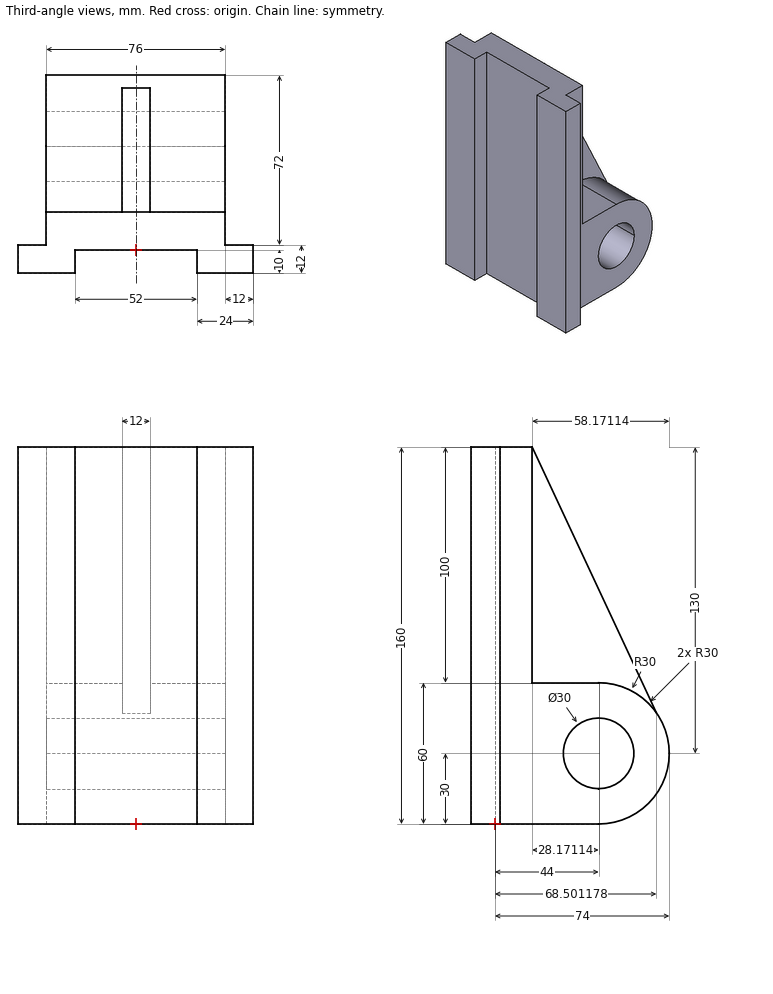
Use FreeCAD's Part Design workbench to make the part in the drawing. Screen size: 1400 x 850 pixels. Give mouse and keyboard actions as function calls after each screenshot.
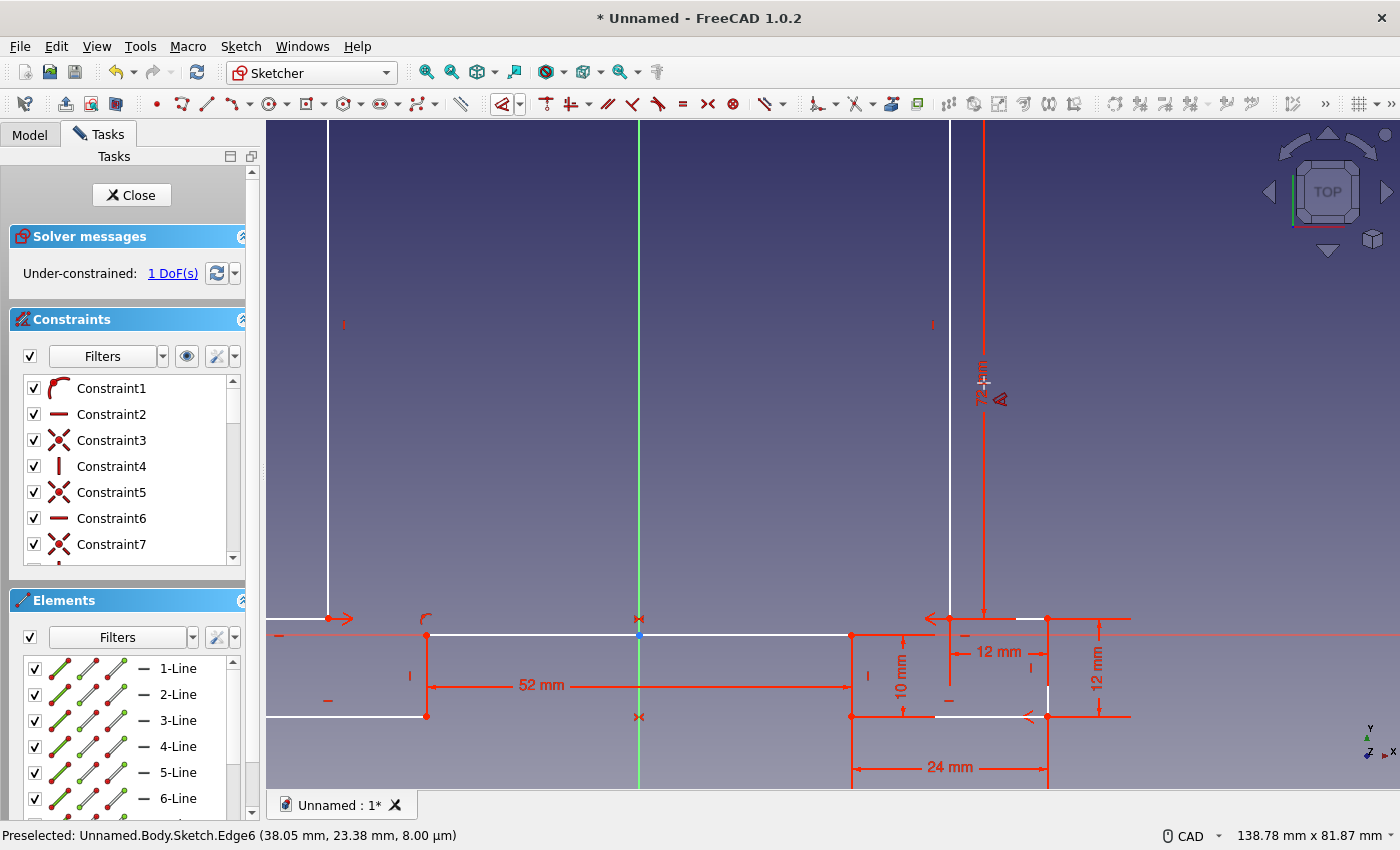
scroll(1020, 619, down, 2)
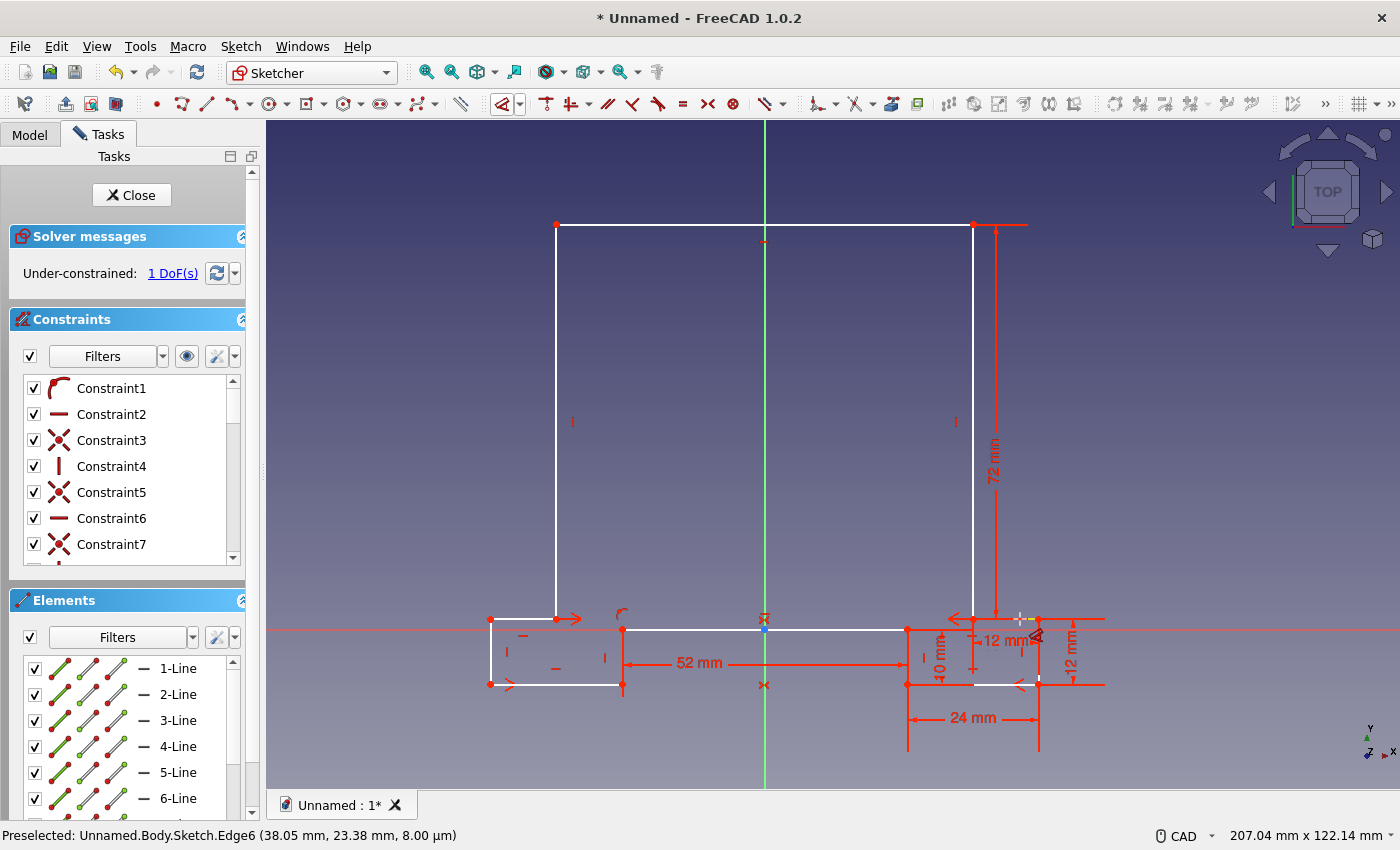
click(848, 225)
click(669, 191)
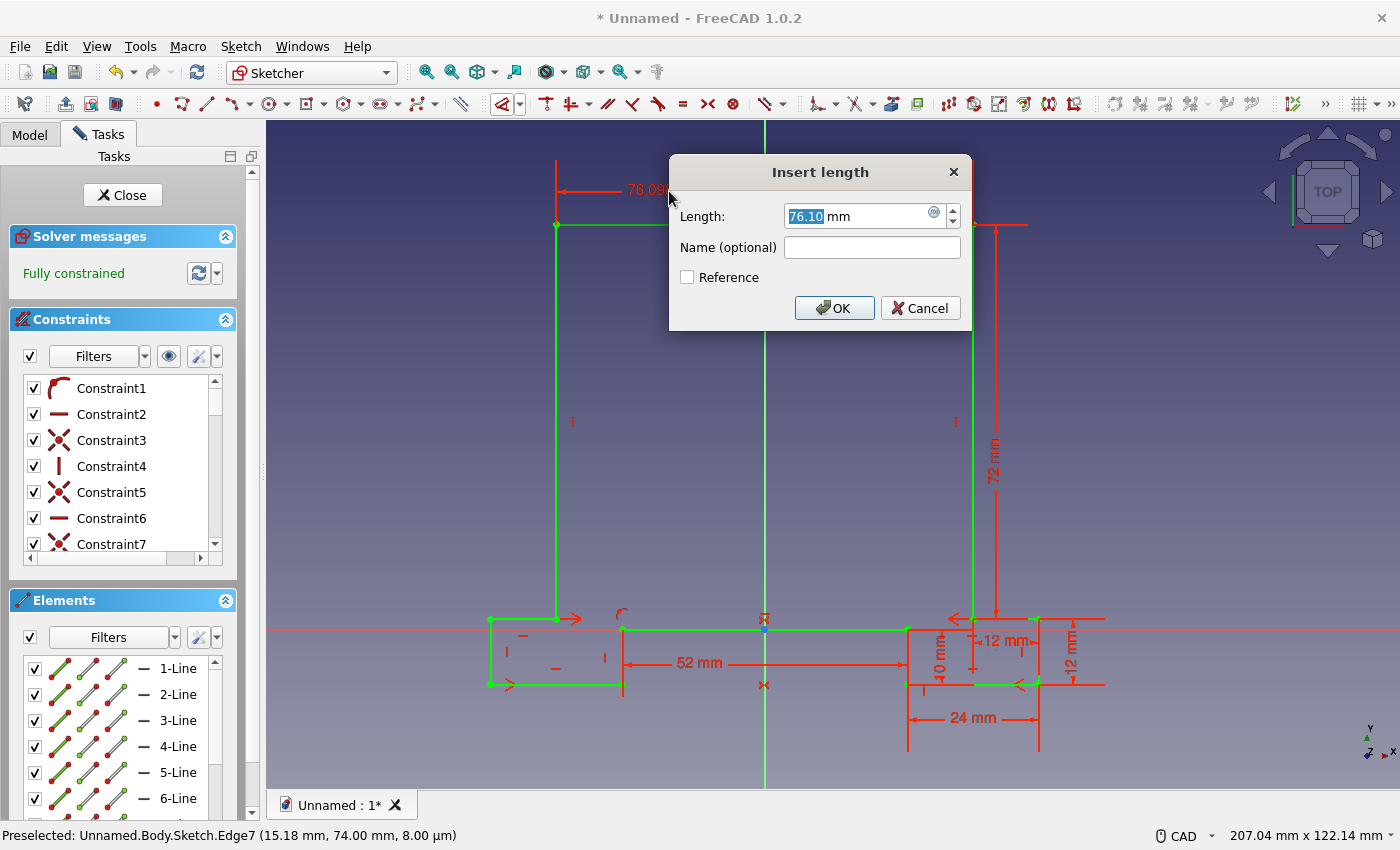
text(76)
key(Return)
key(Escape)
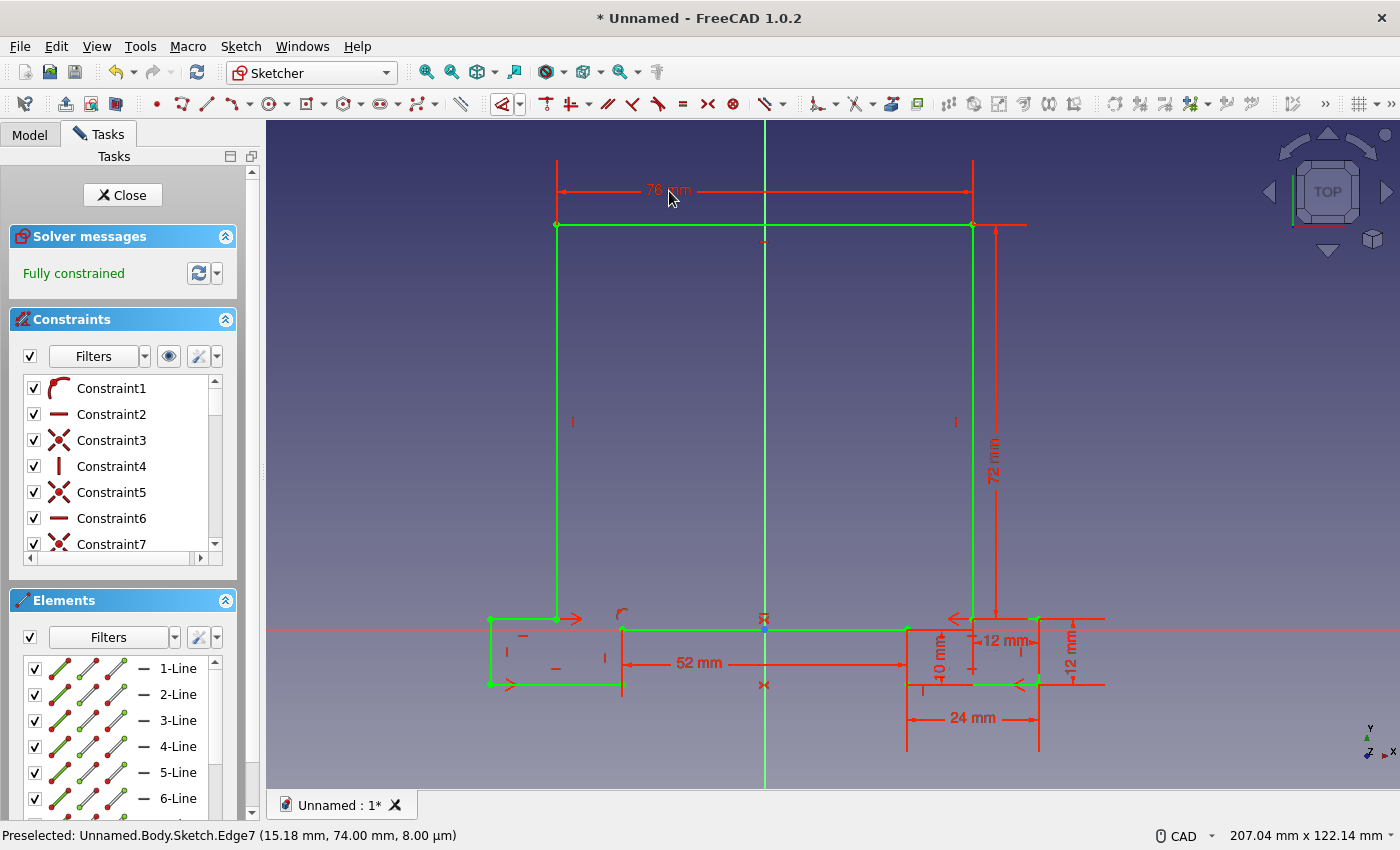
click(123, 195)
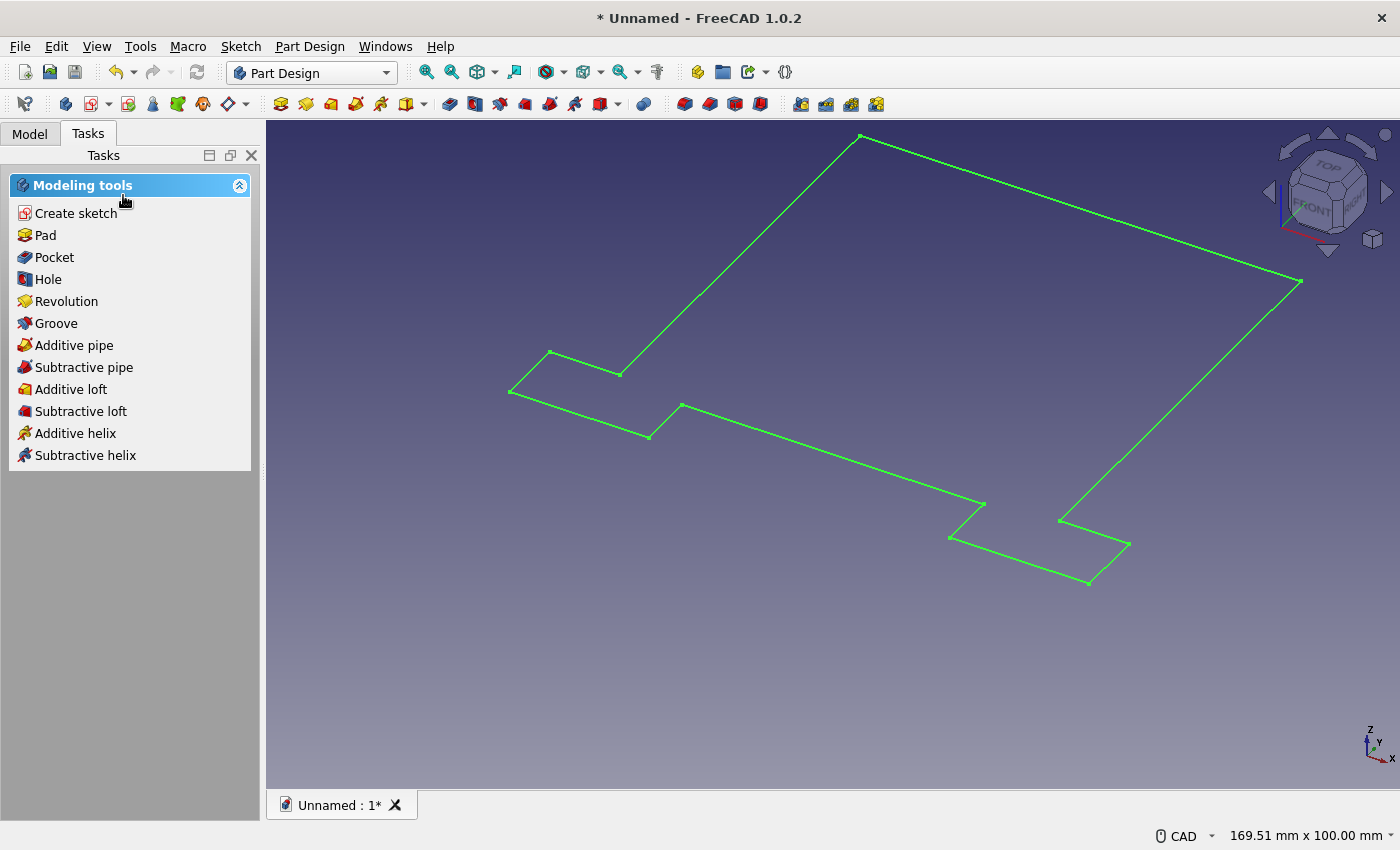
click(281, 104)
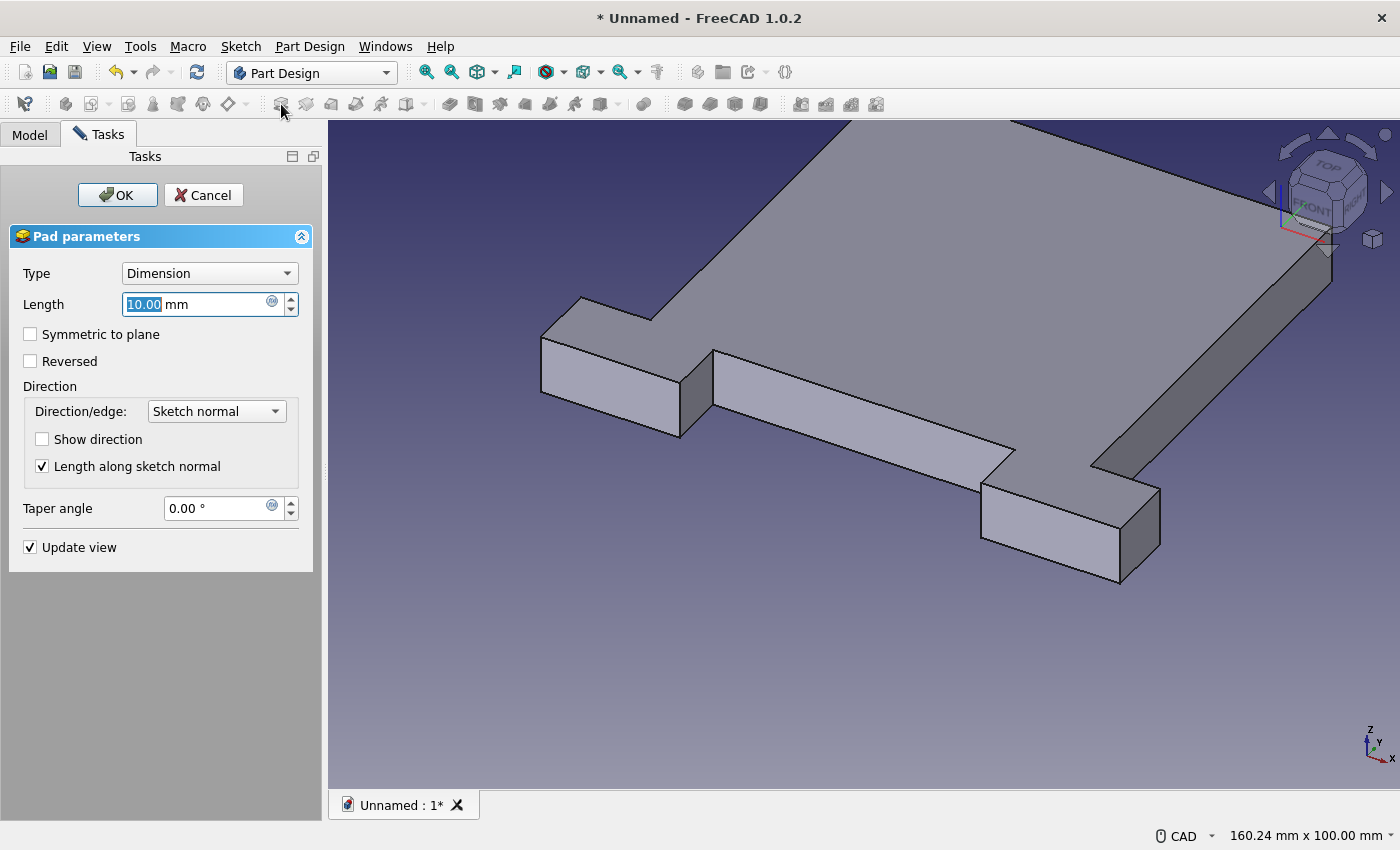
text(160)
key(Tab)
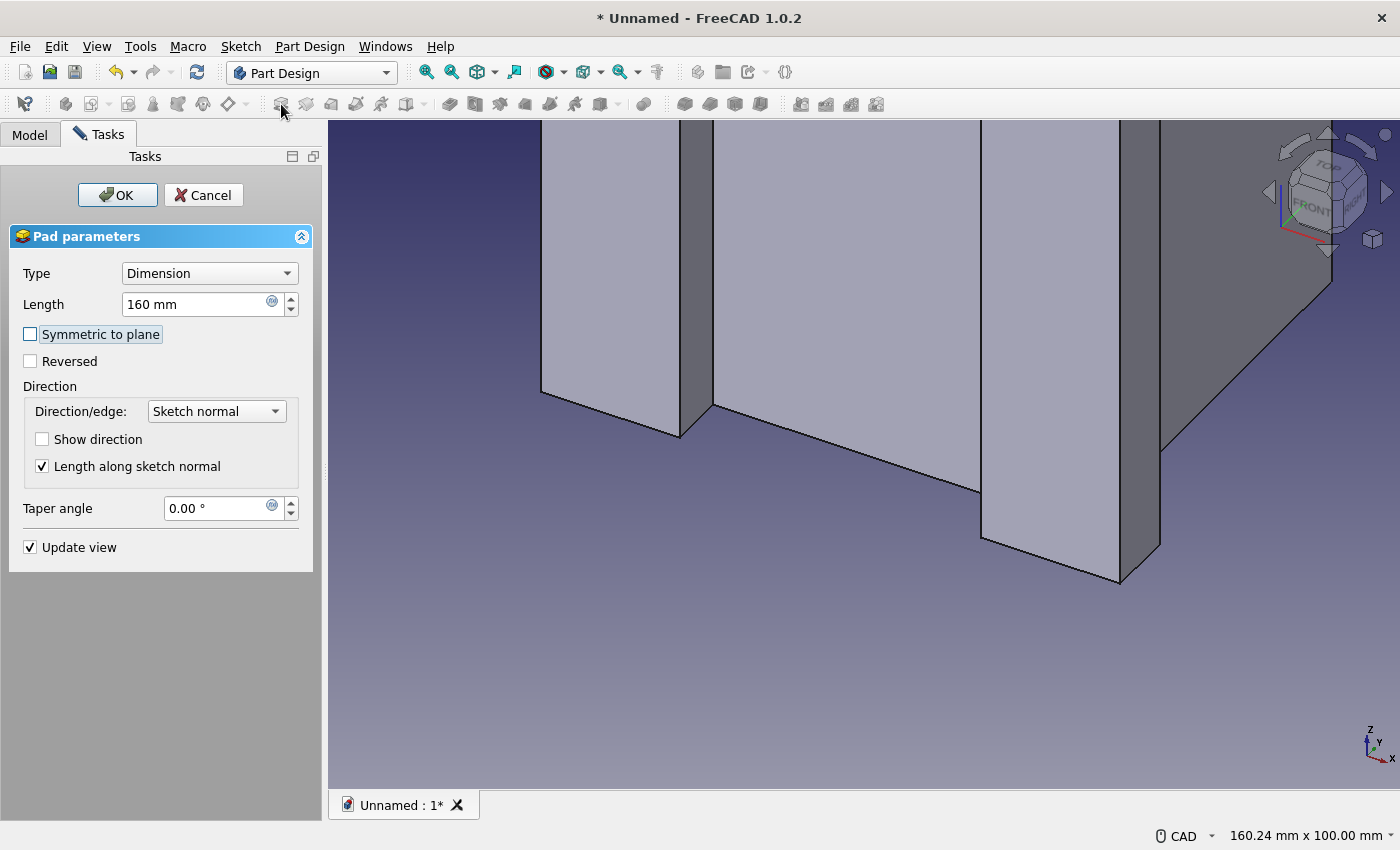
click(118, 195)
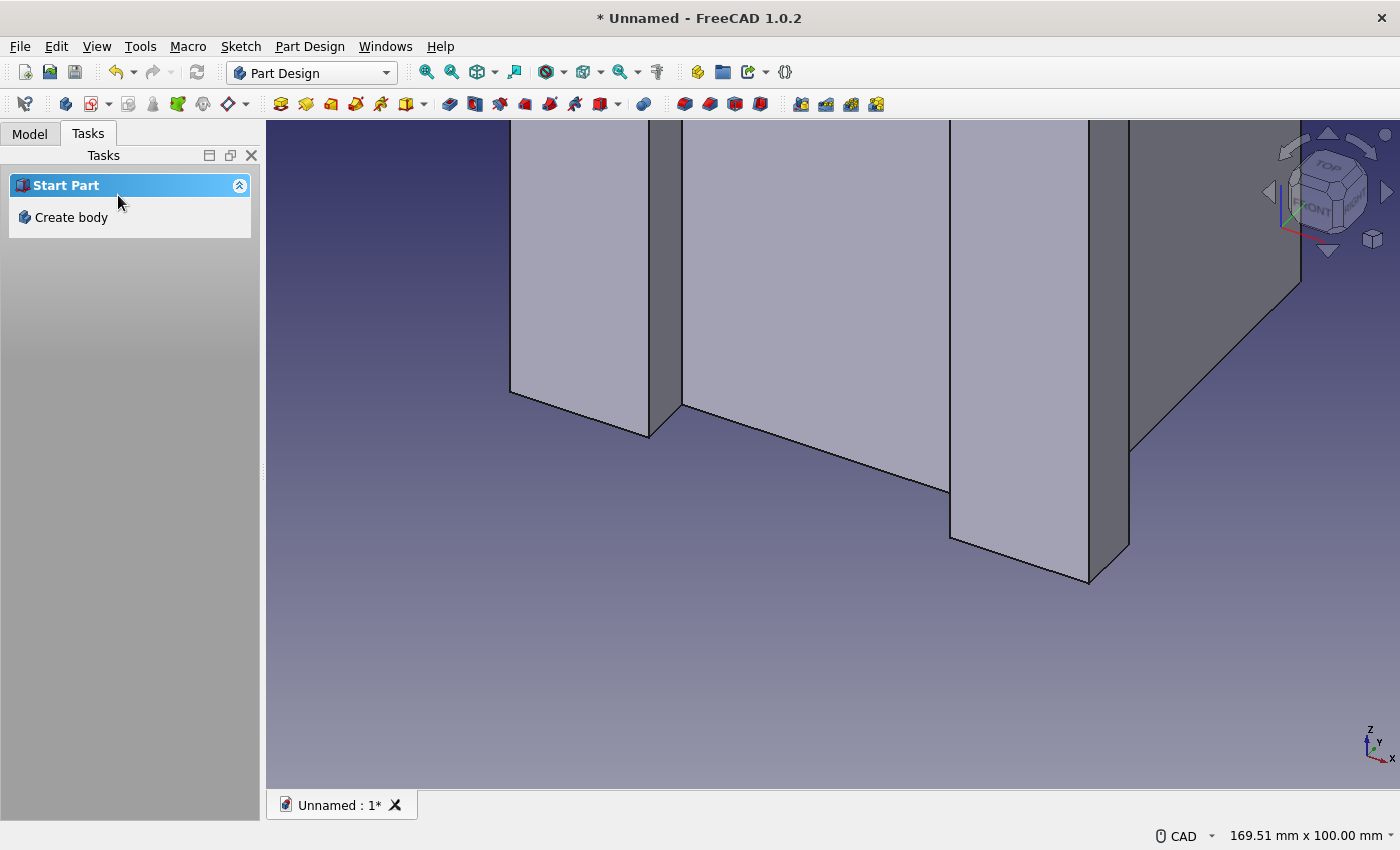
key(v)
key(f)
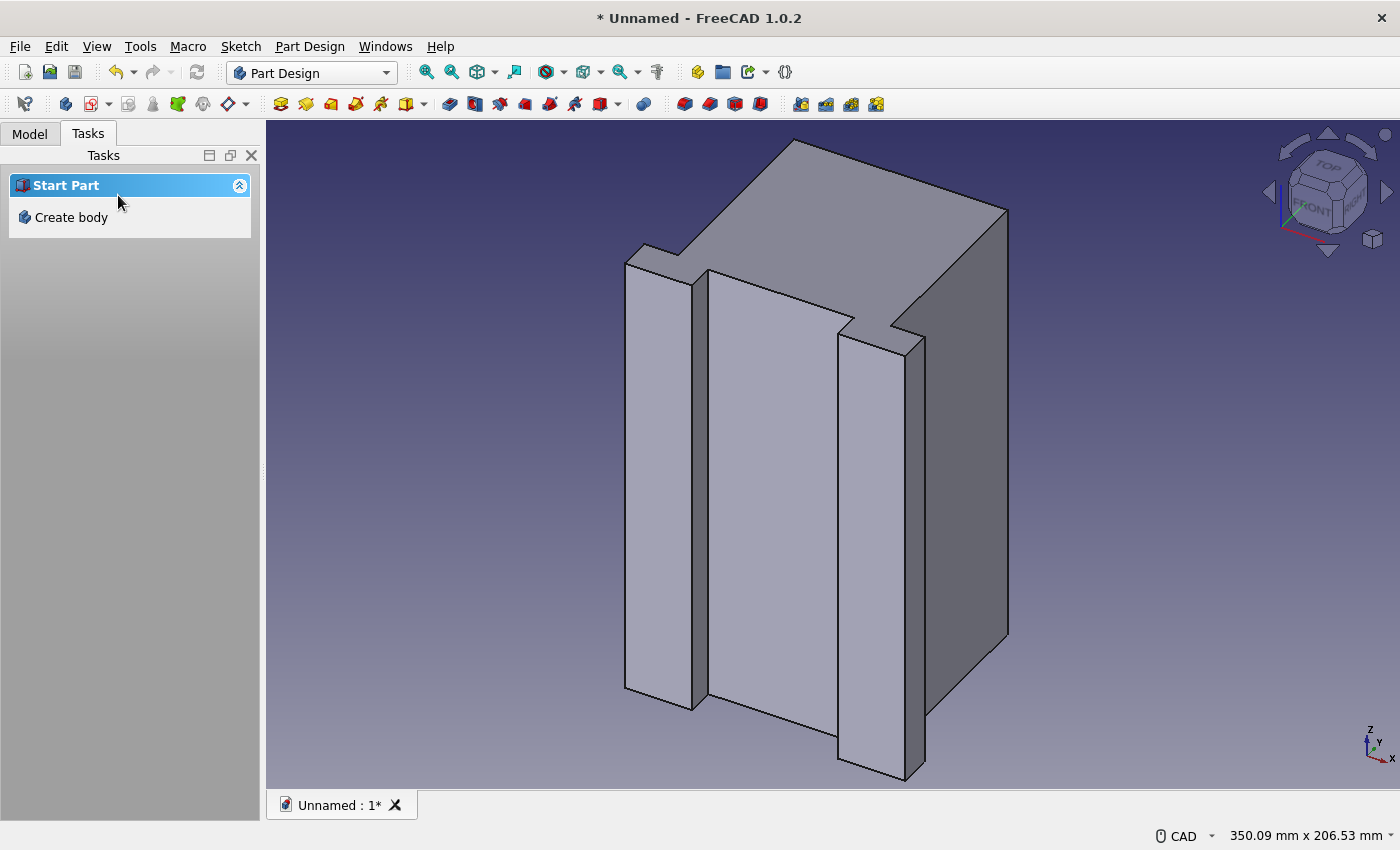
click(949, 418)